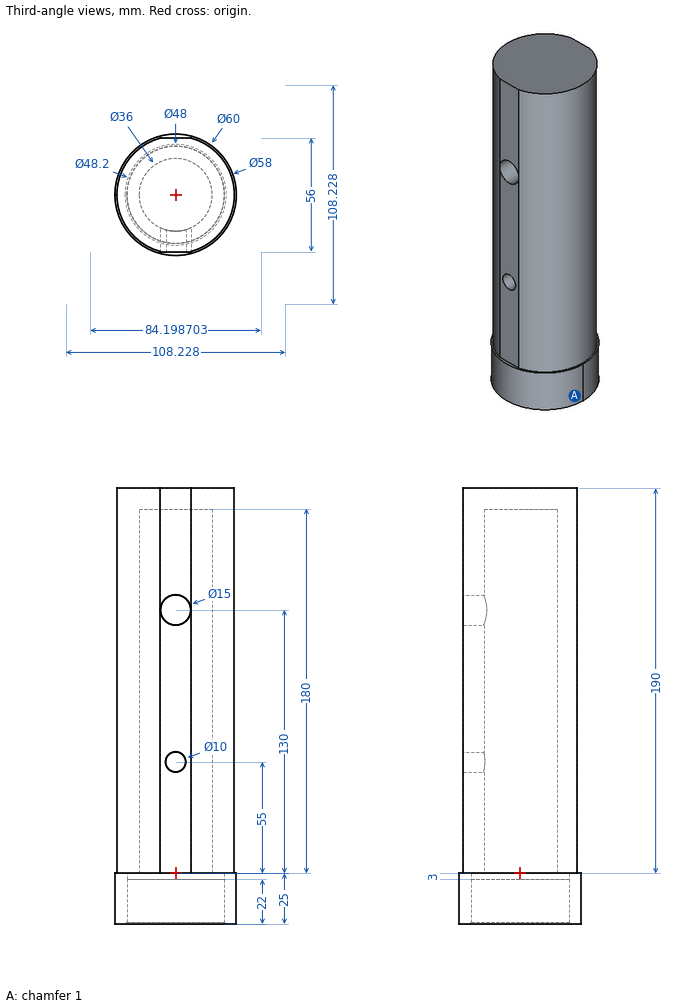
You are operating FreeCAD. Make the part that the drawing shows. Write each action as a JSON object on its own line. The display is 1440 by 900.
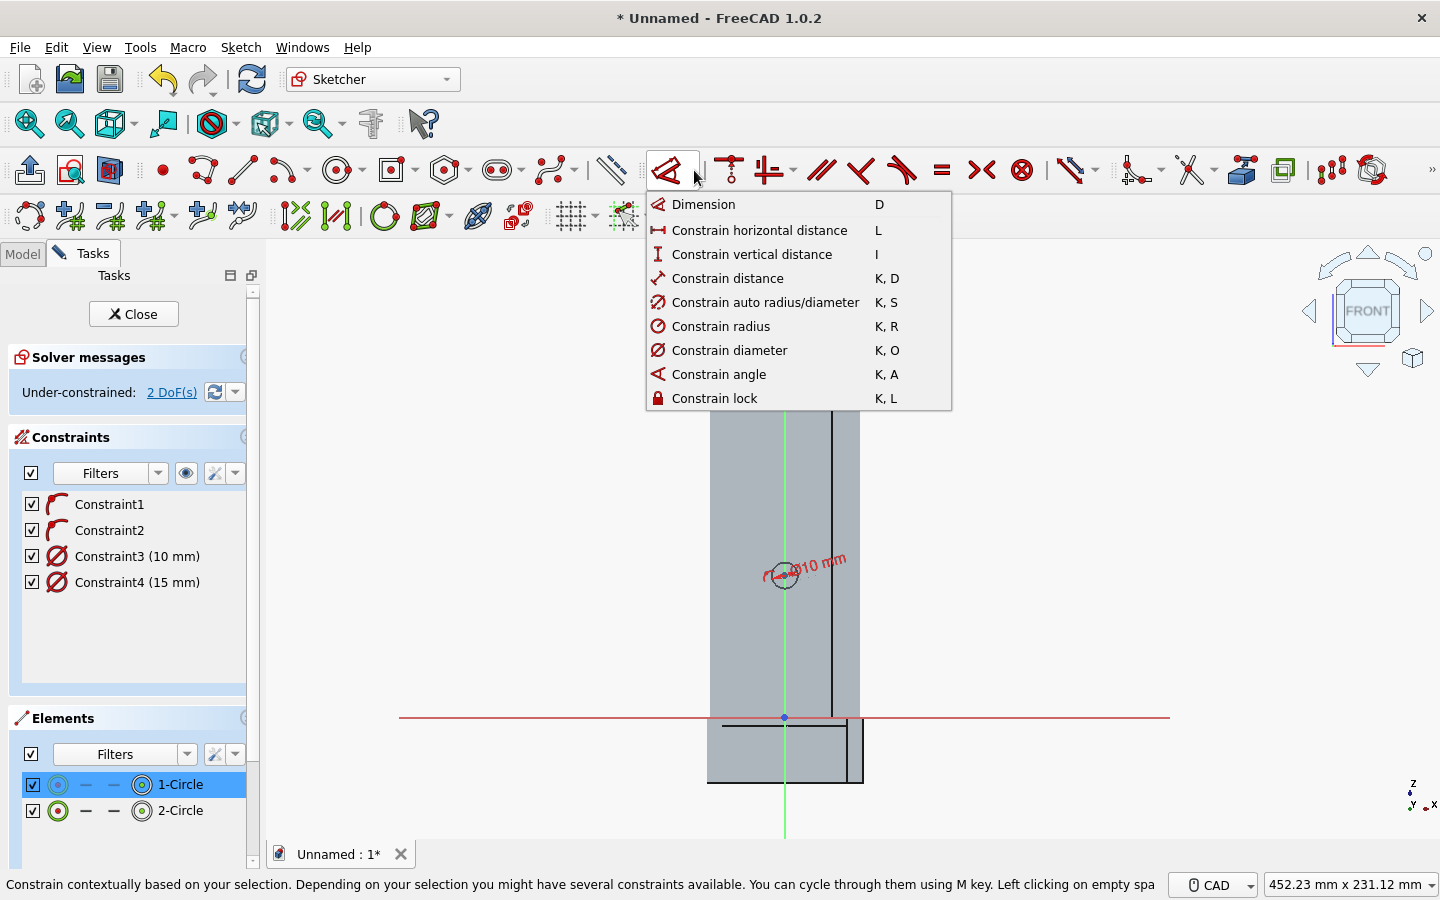
{"action": "left_click", "coordinate": [799, 254]}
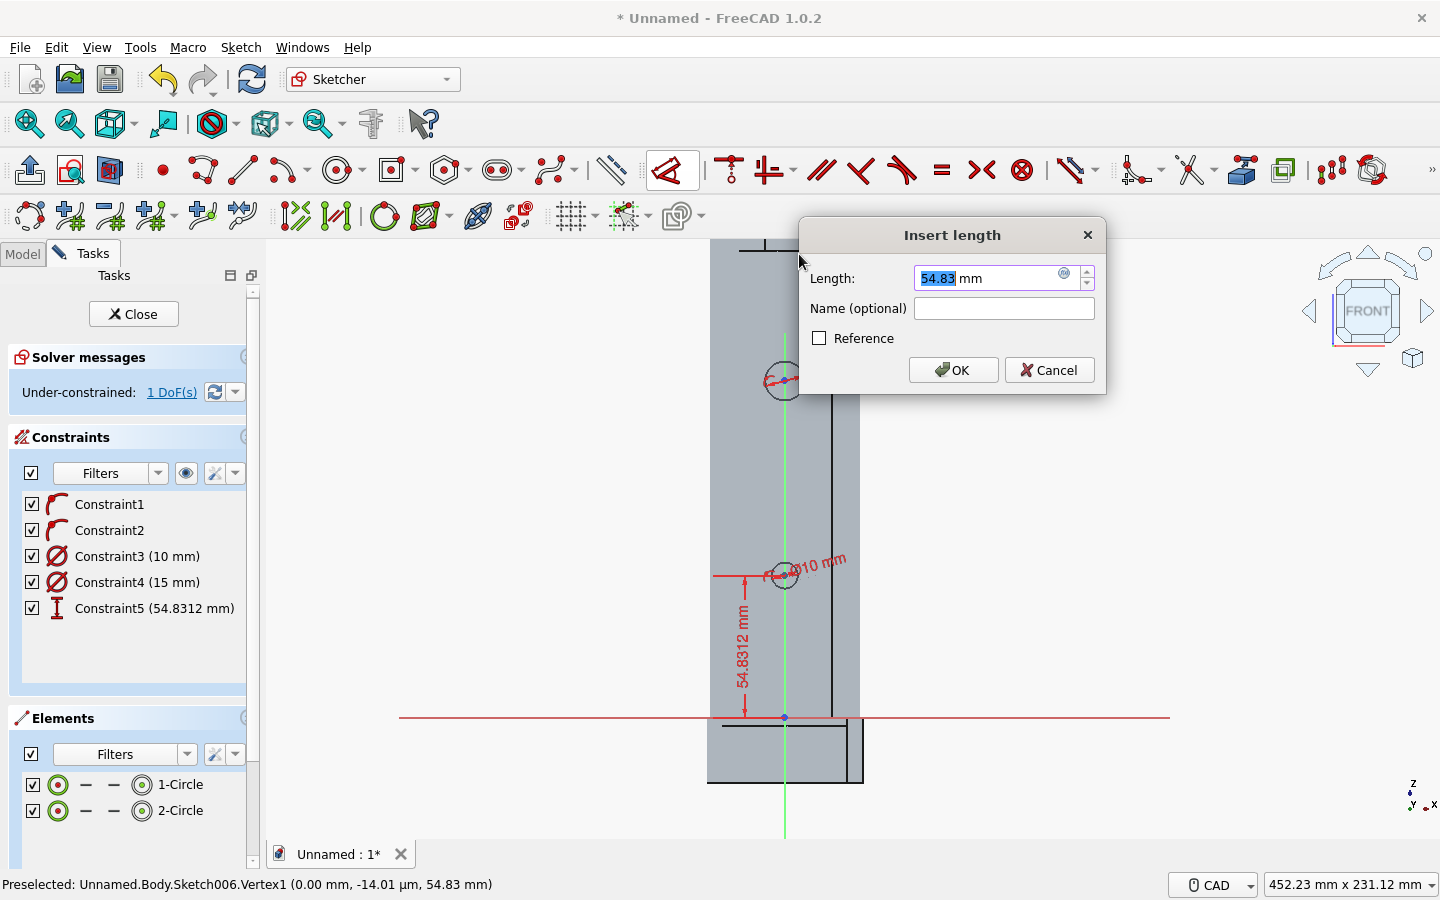
{"action": "type", "text": "55"}
{"action": "key", "text": "Return"}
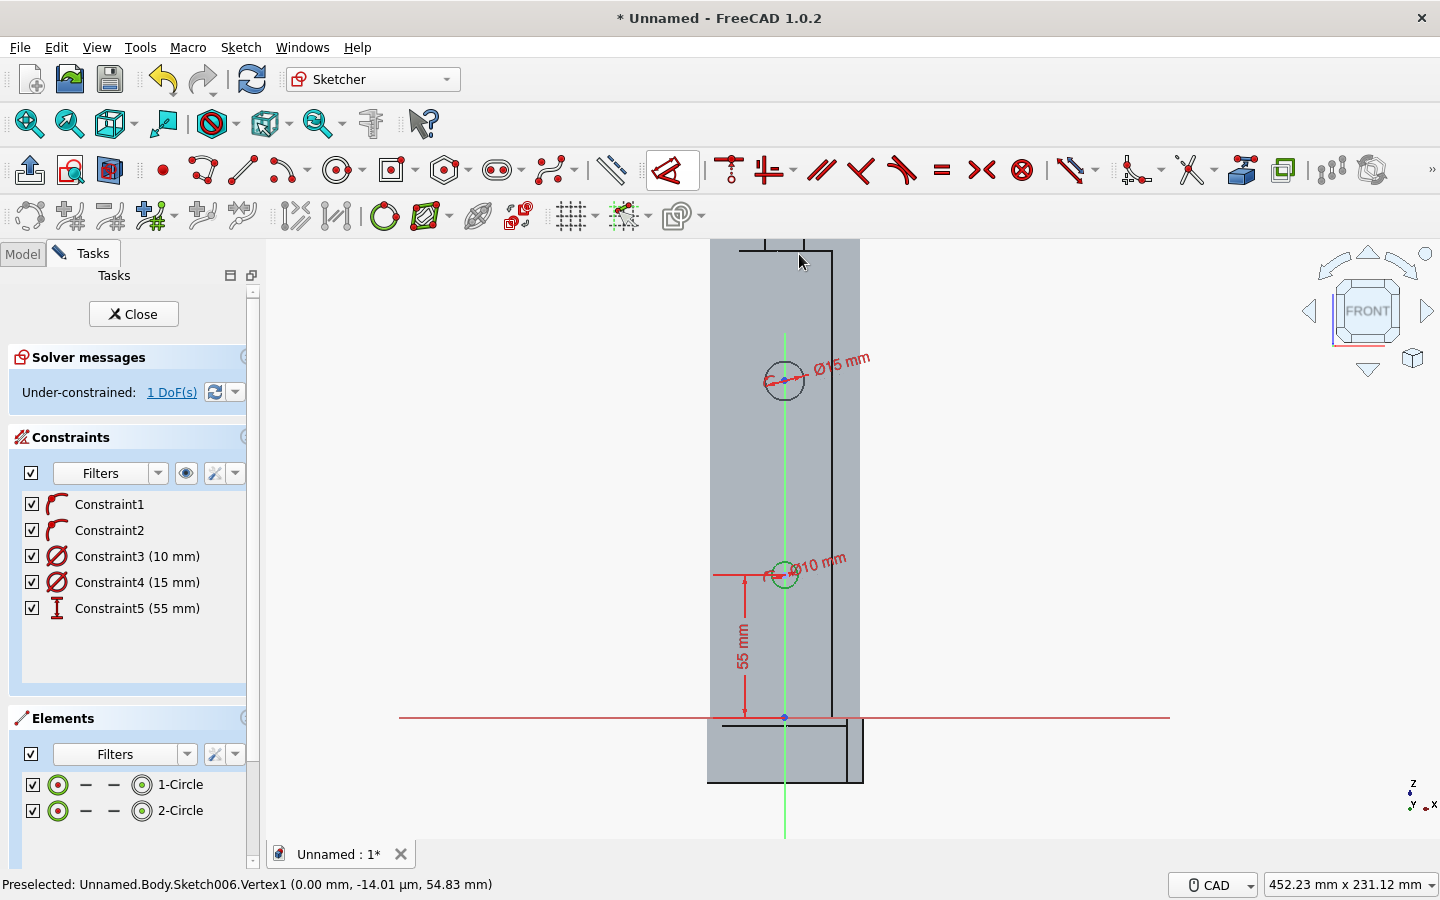
{"action": "left_click", "coordinate": [785, 381]}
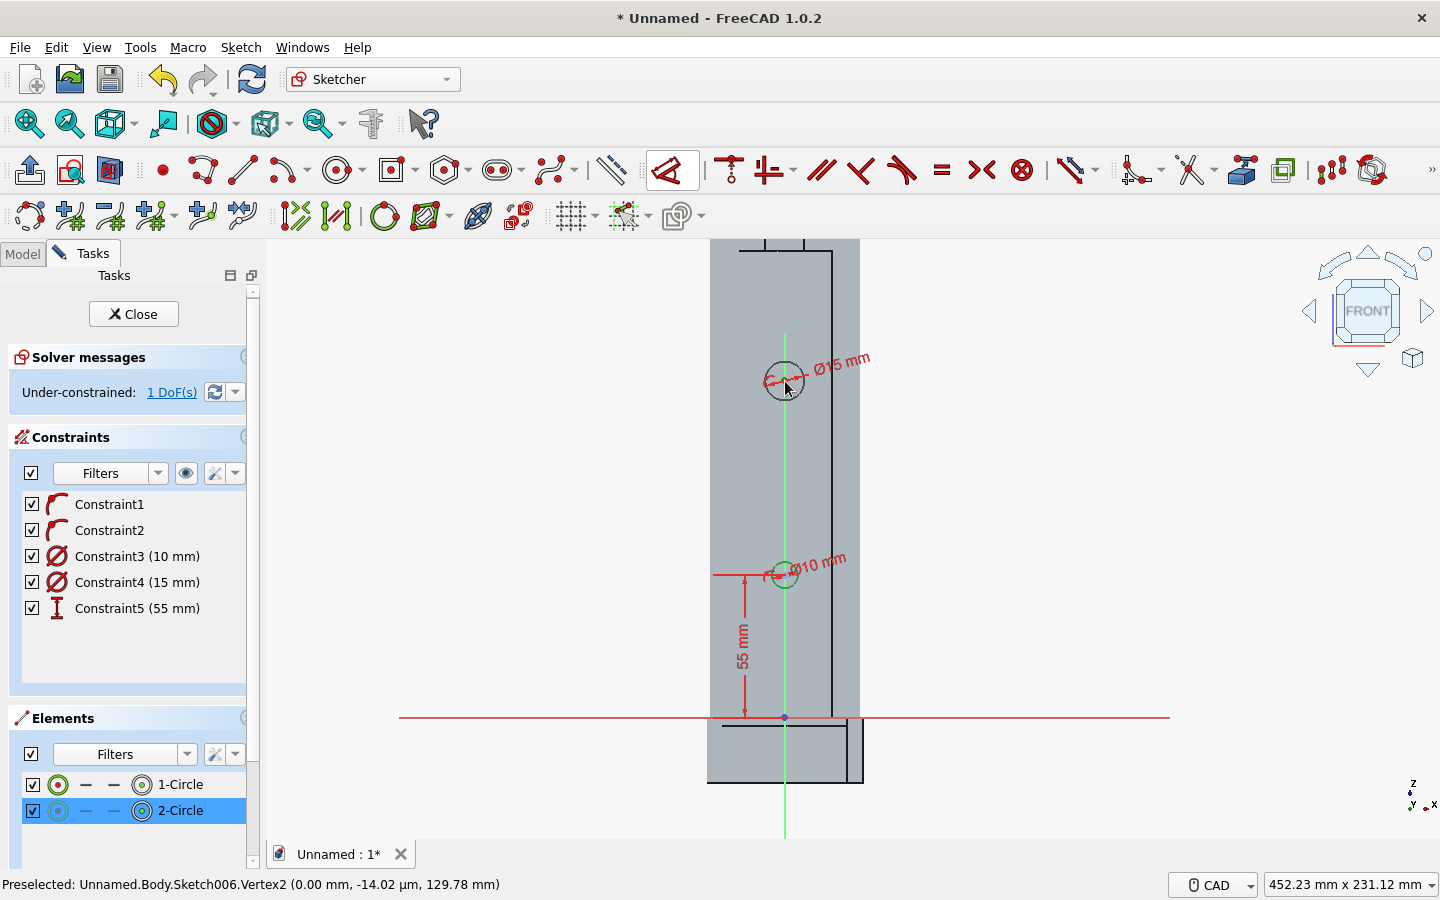
{"action": "left_click", "coordinate": [694, 170]}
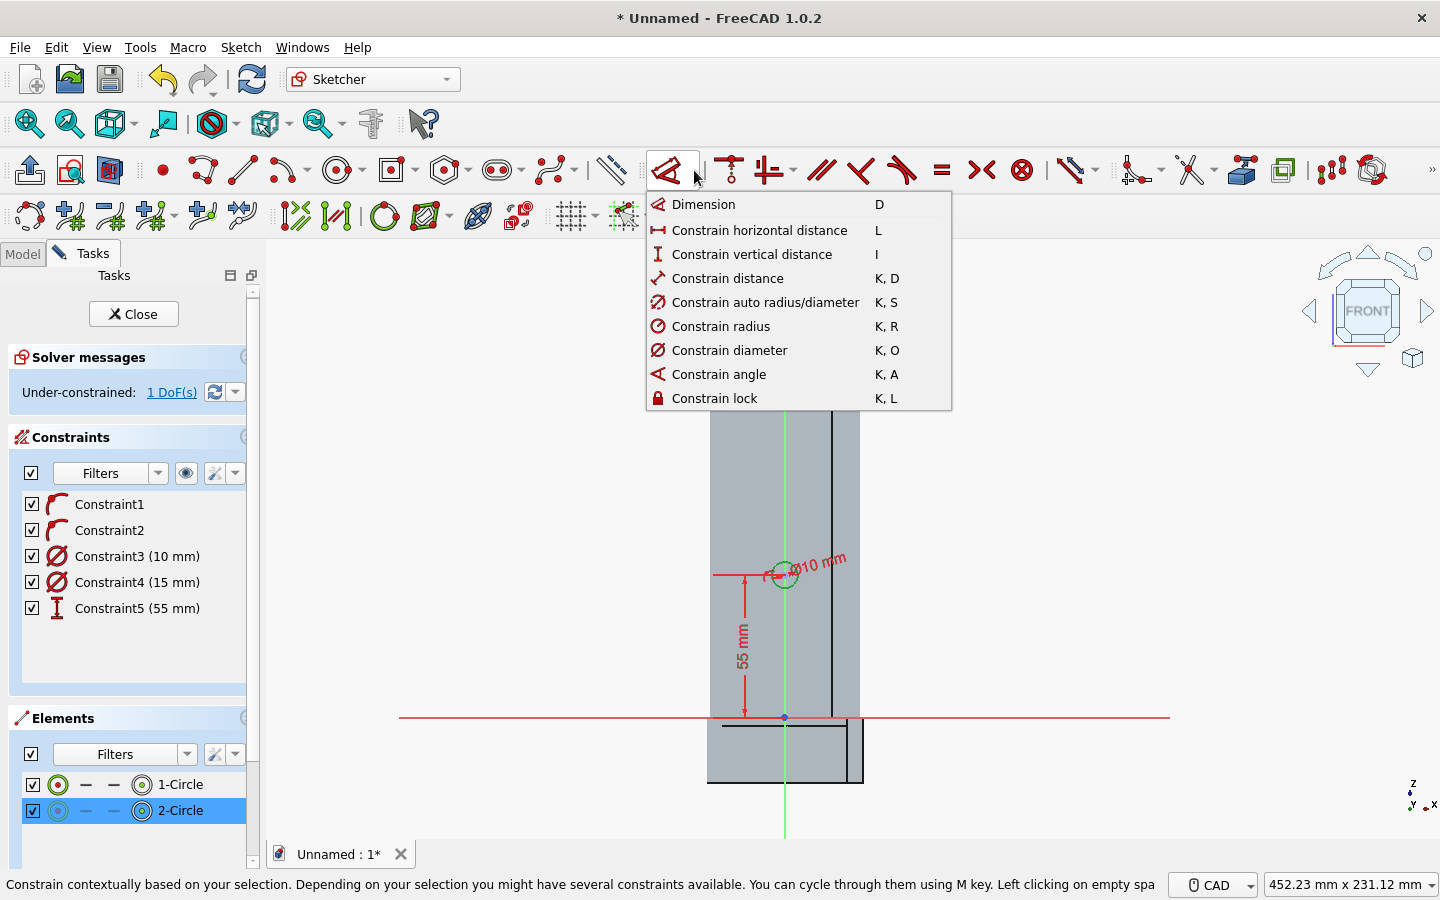
{"action": "left_click", "coordinate": [799, 254]}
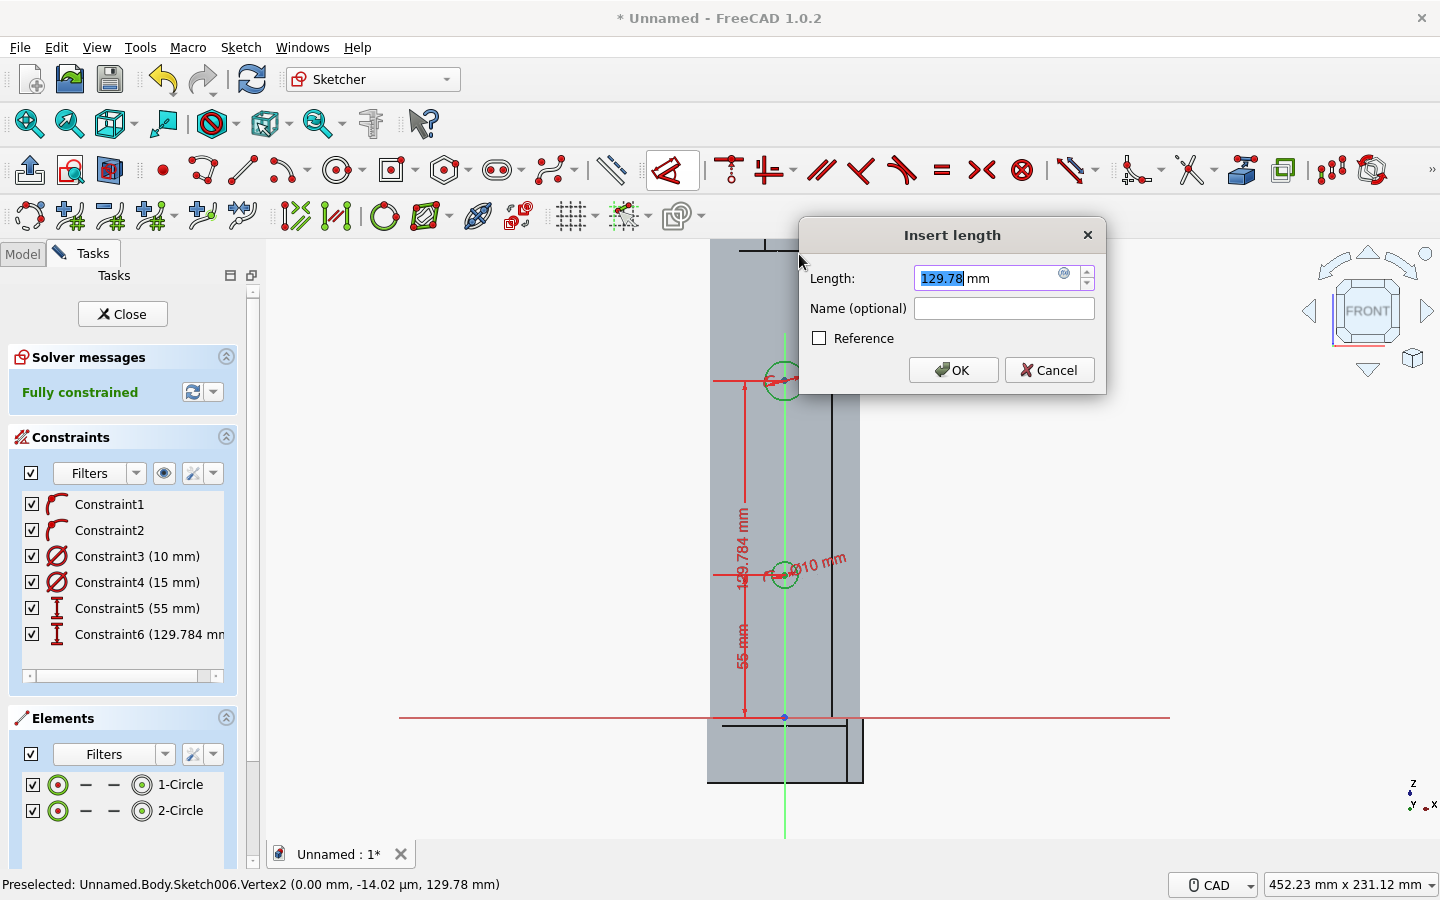
{"action": "type", "text": "130"}
{"action": "key", "text": "Return"}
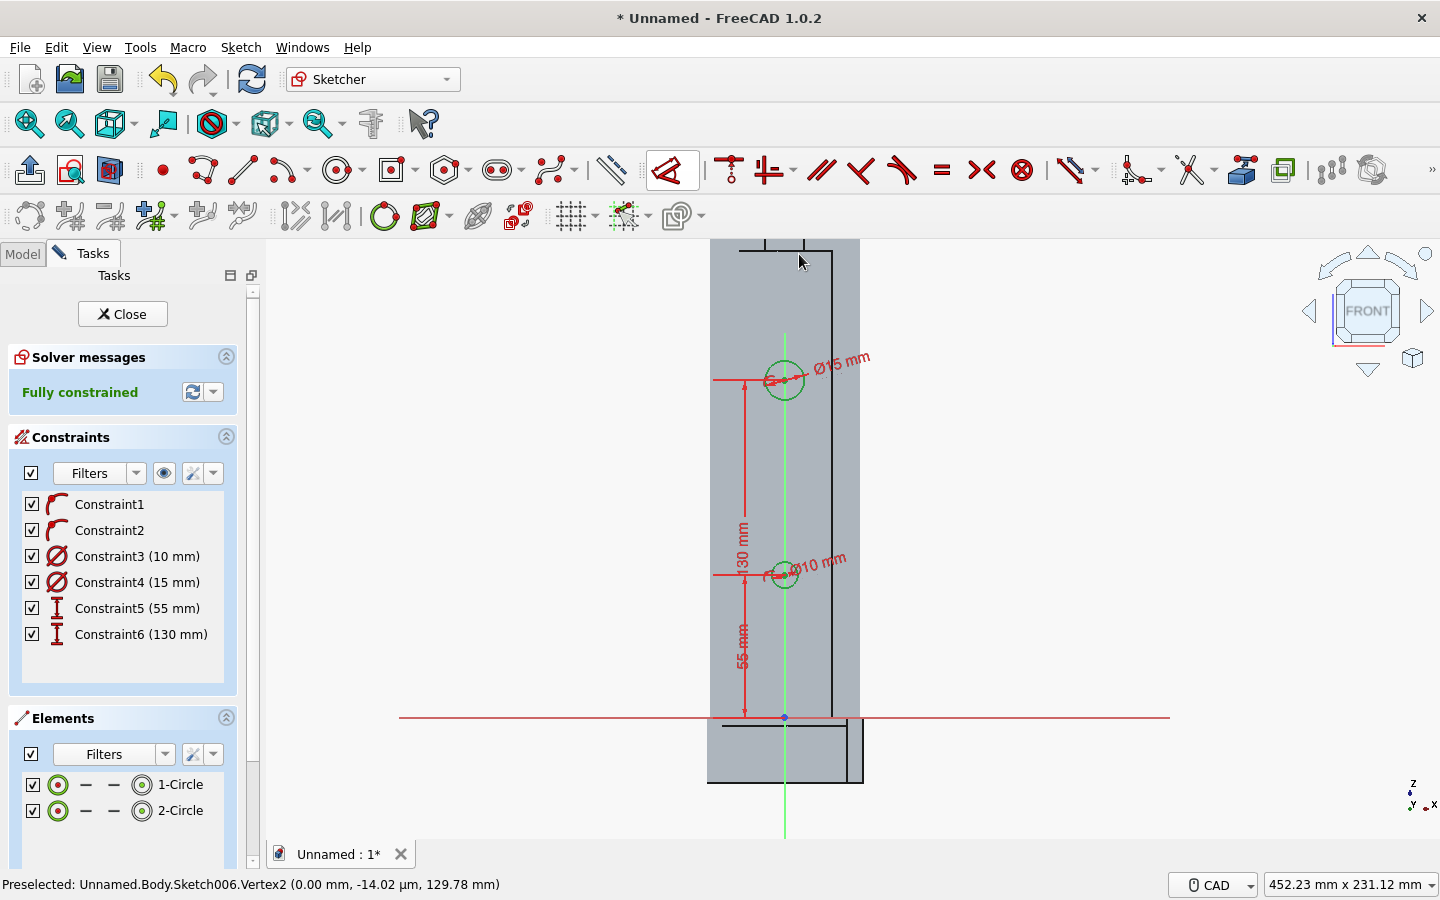
{"action": "left_click", "coordinate": [123, 314]}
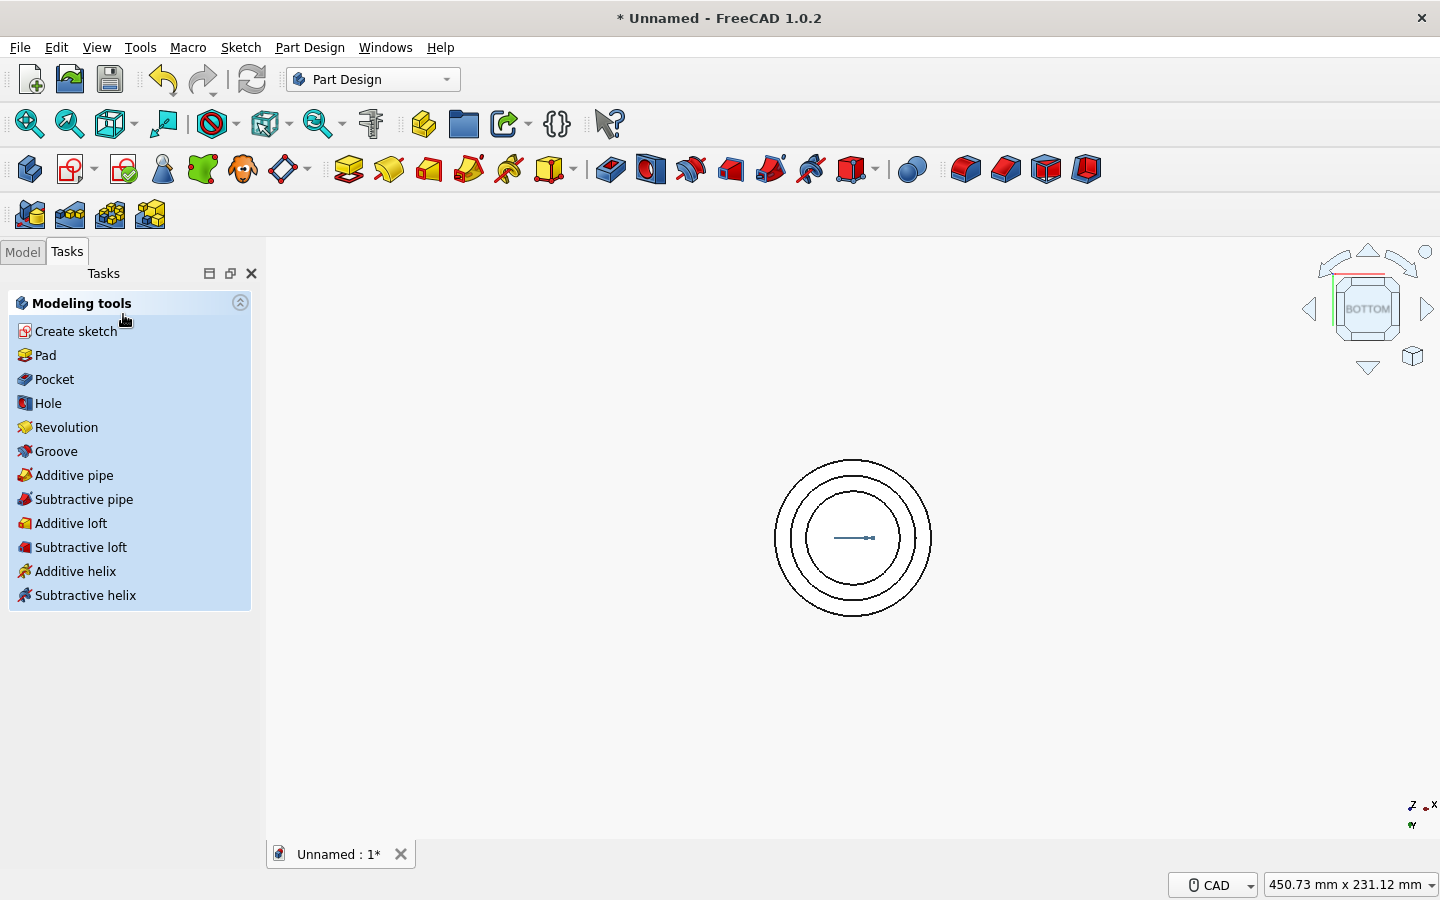
{"action": "left_click", "coordinate": [612, 170]}